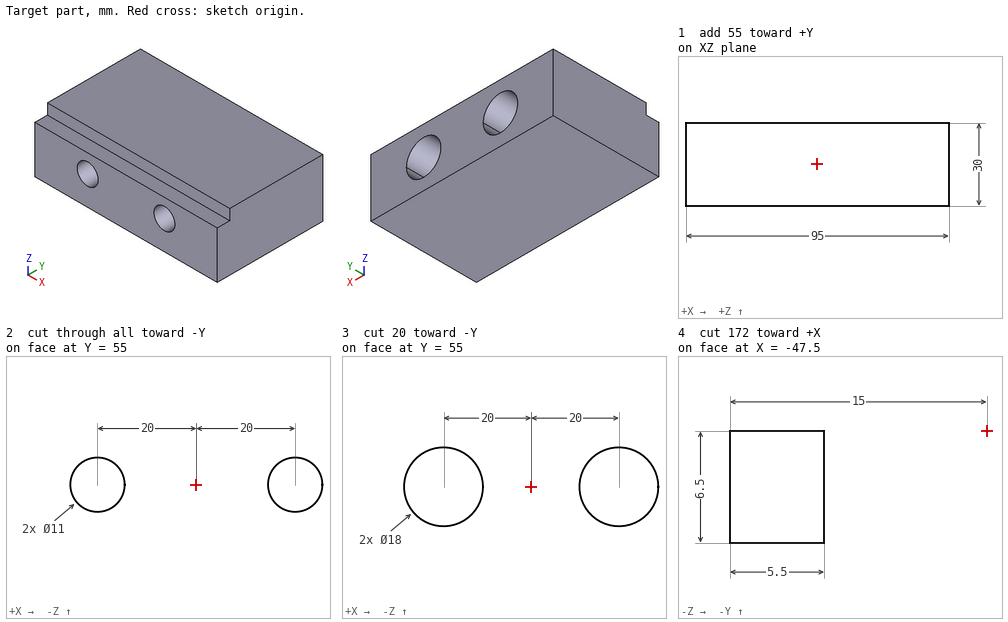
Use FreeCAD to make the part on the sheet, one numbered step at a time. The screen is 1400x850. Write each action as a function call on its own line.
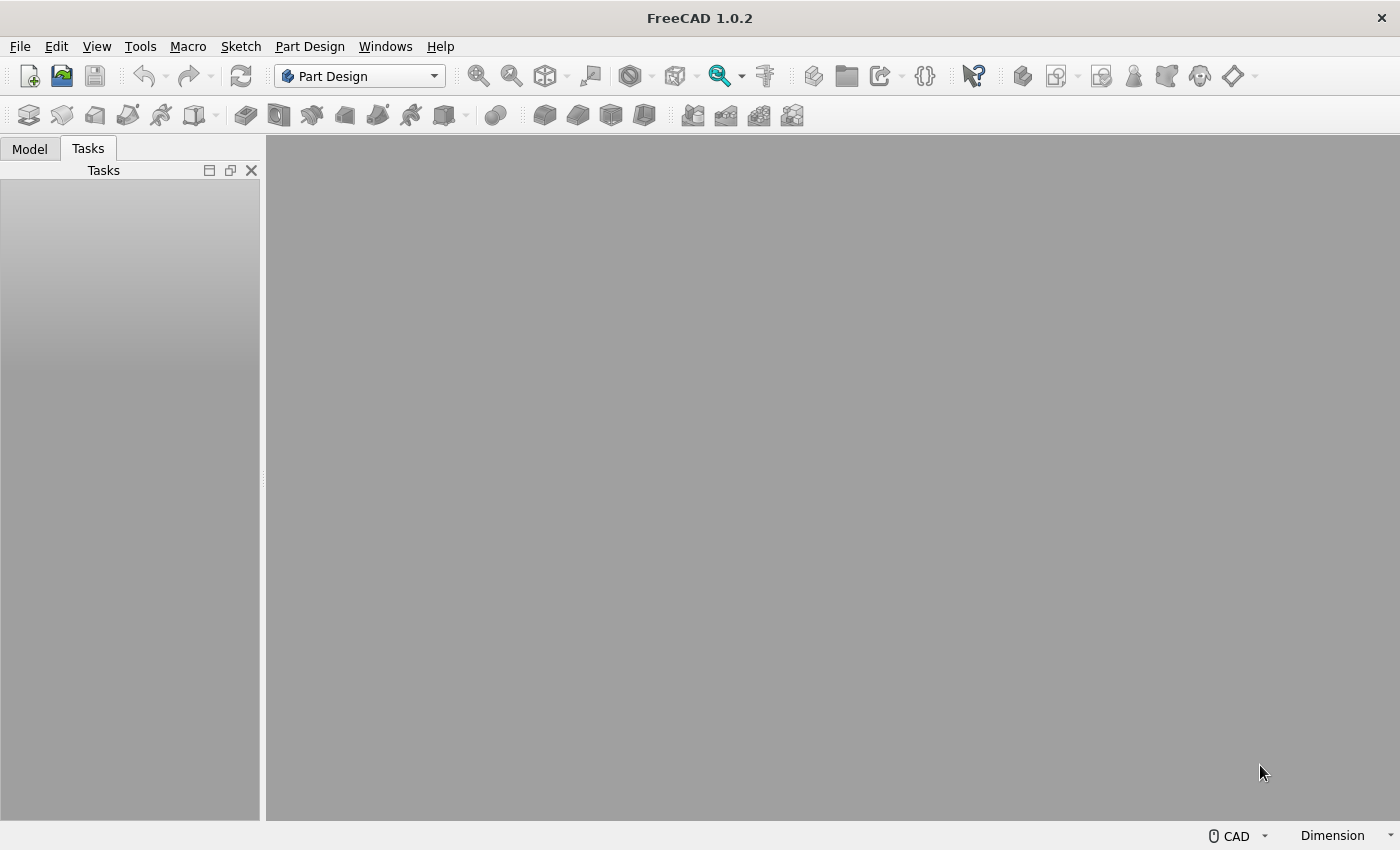
click(29, 76)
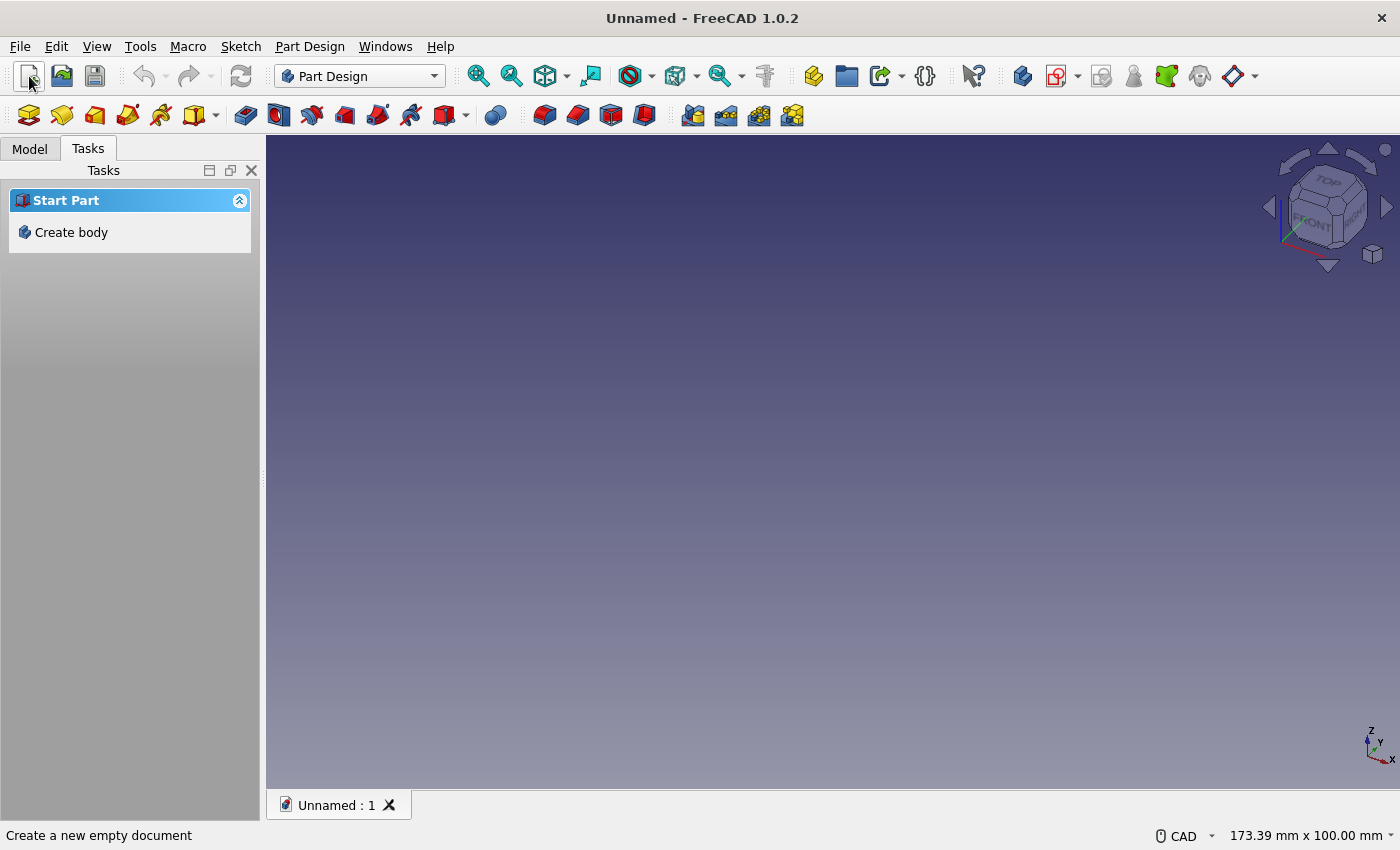
click(1056, 76)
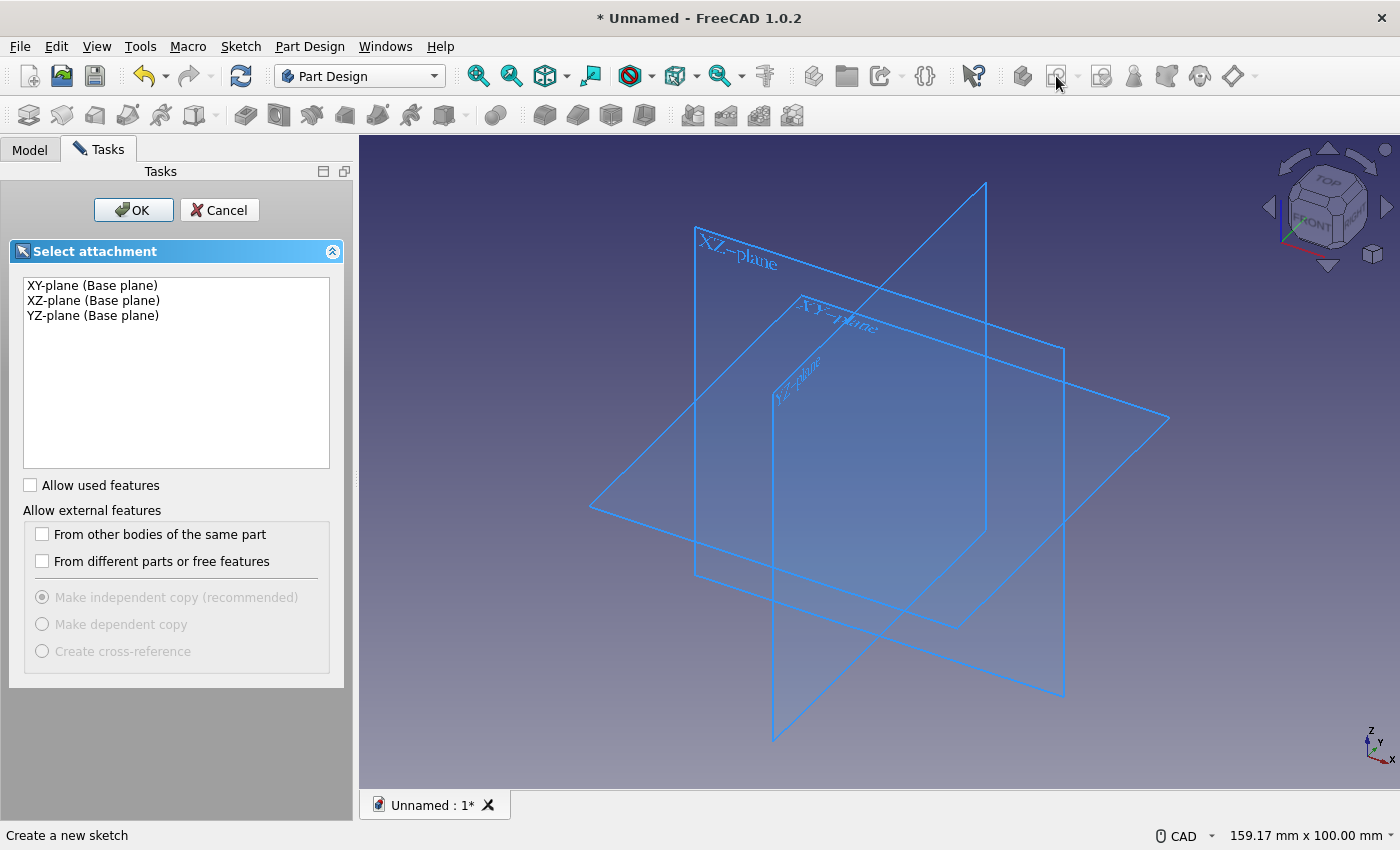
click(84, 300)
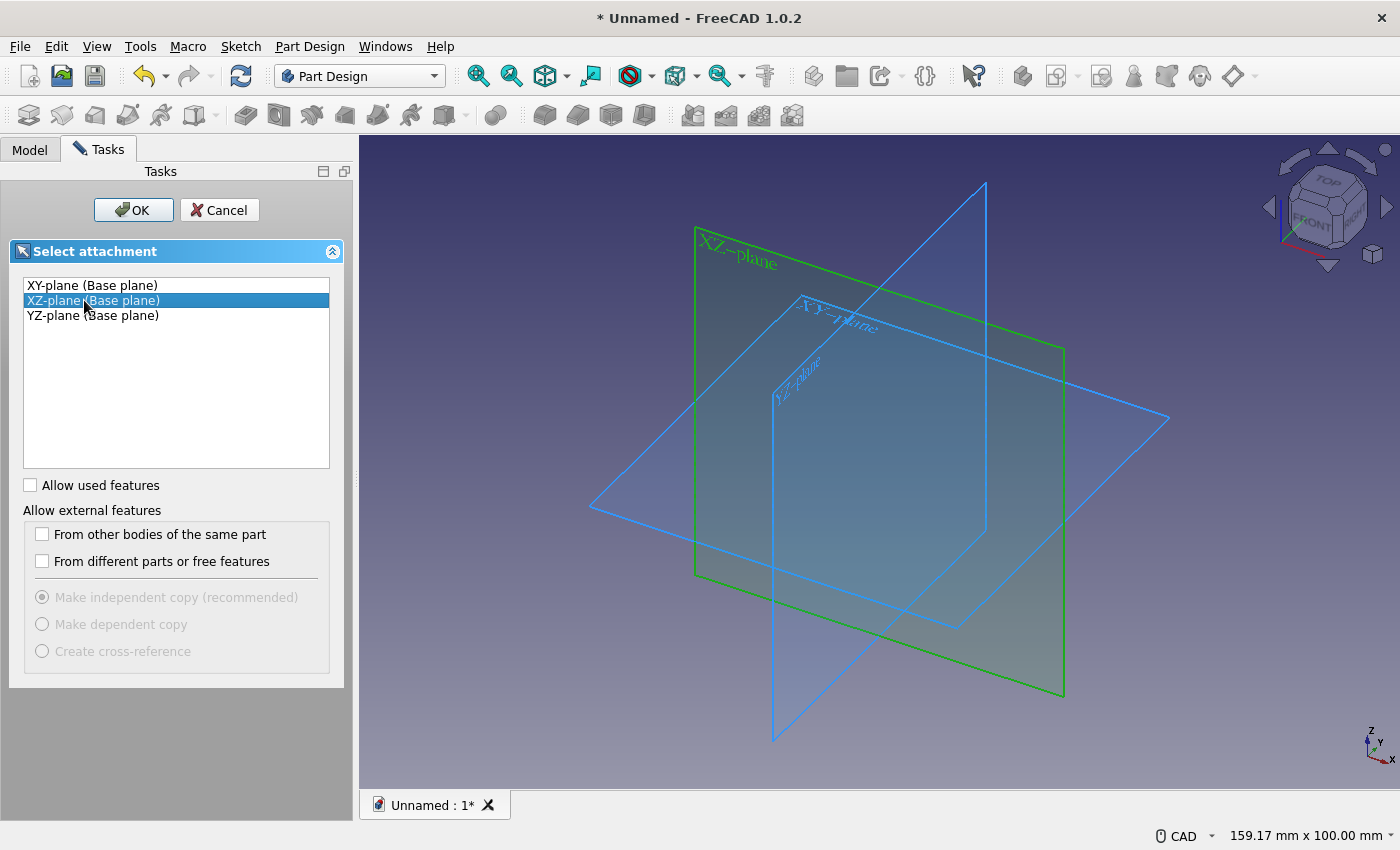
click(134, 210)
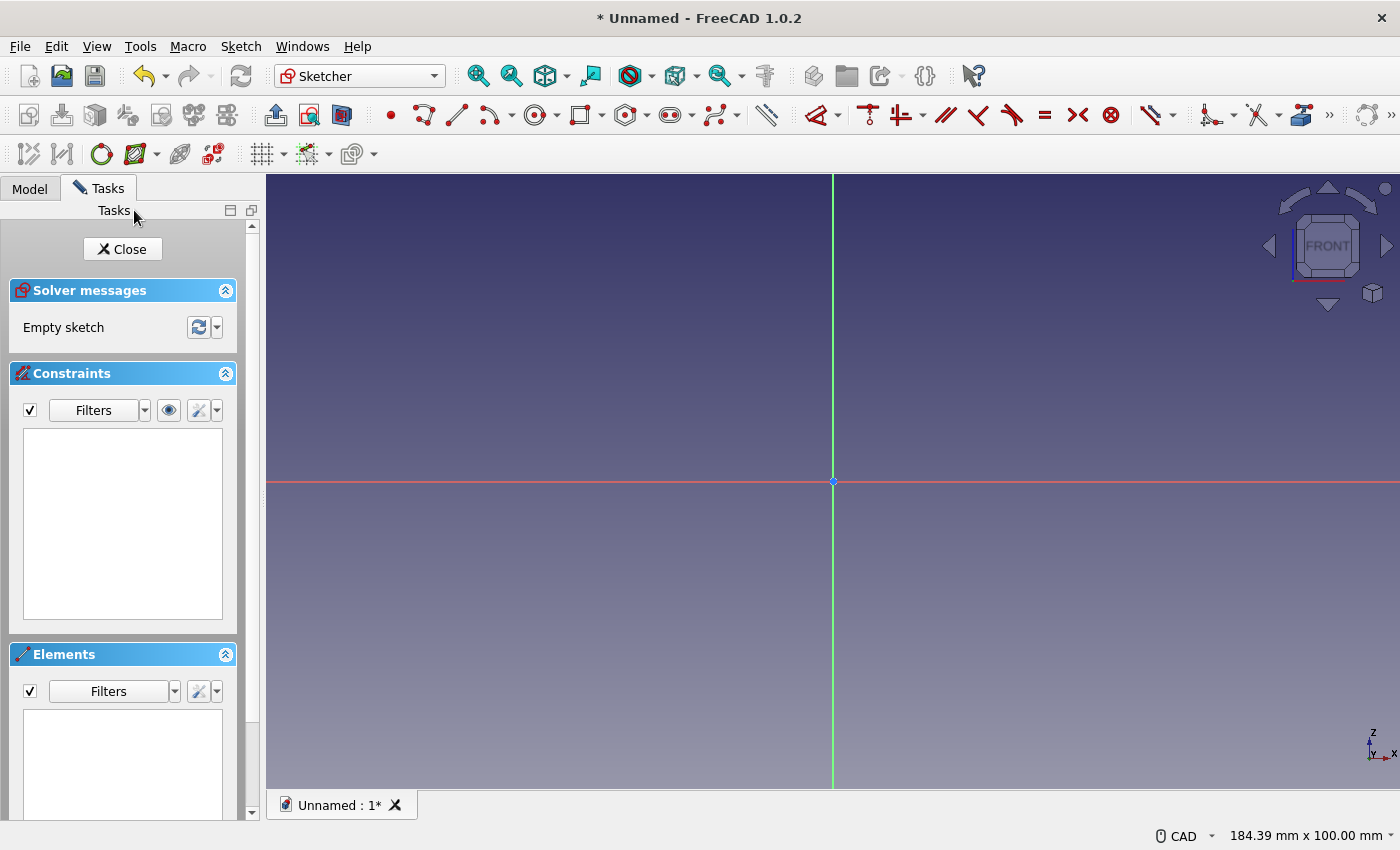
key(g)
key(v)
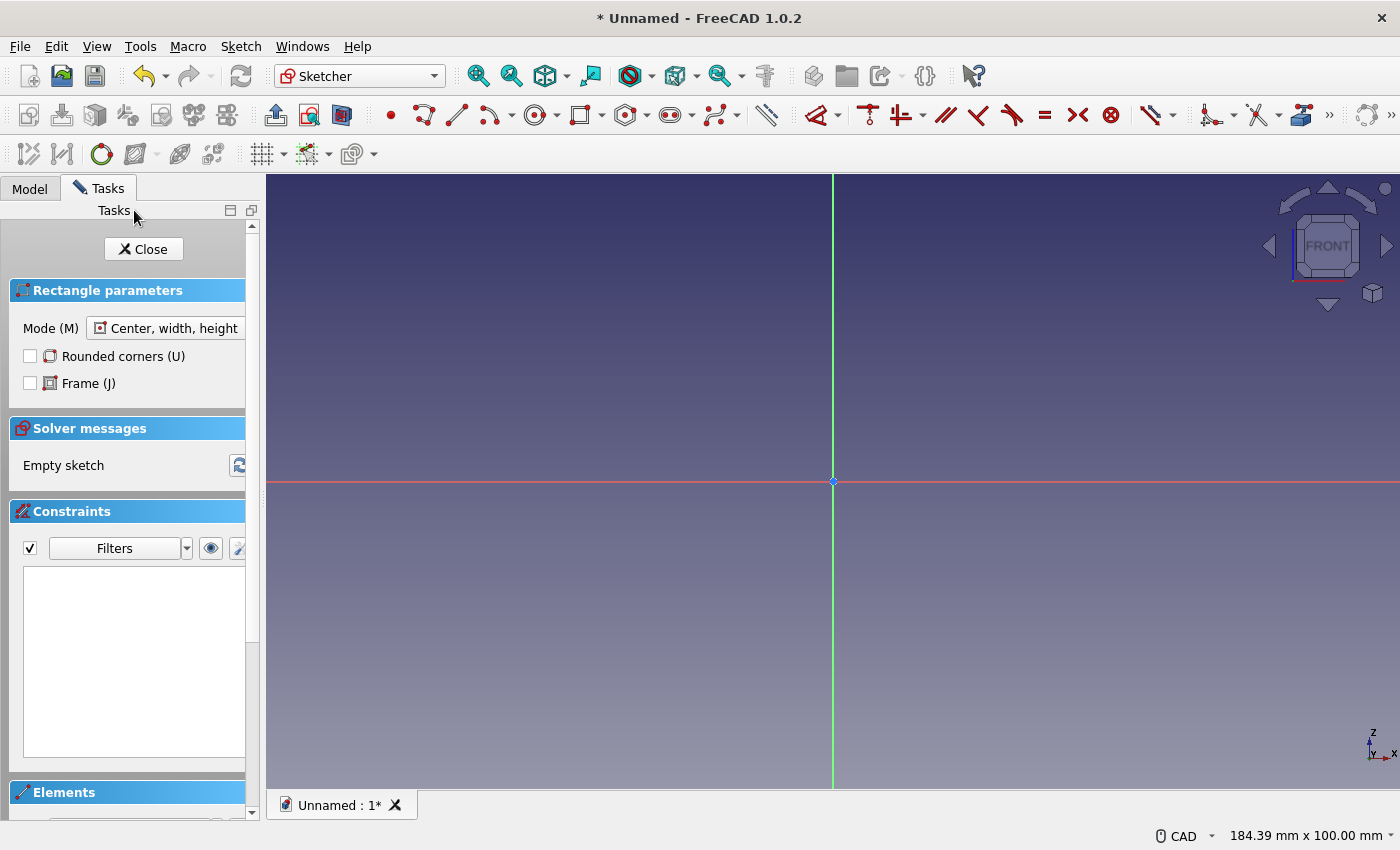
click(833, 482)
move(1125, 389)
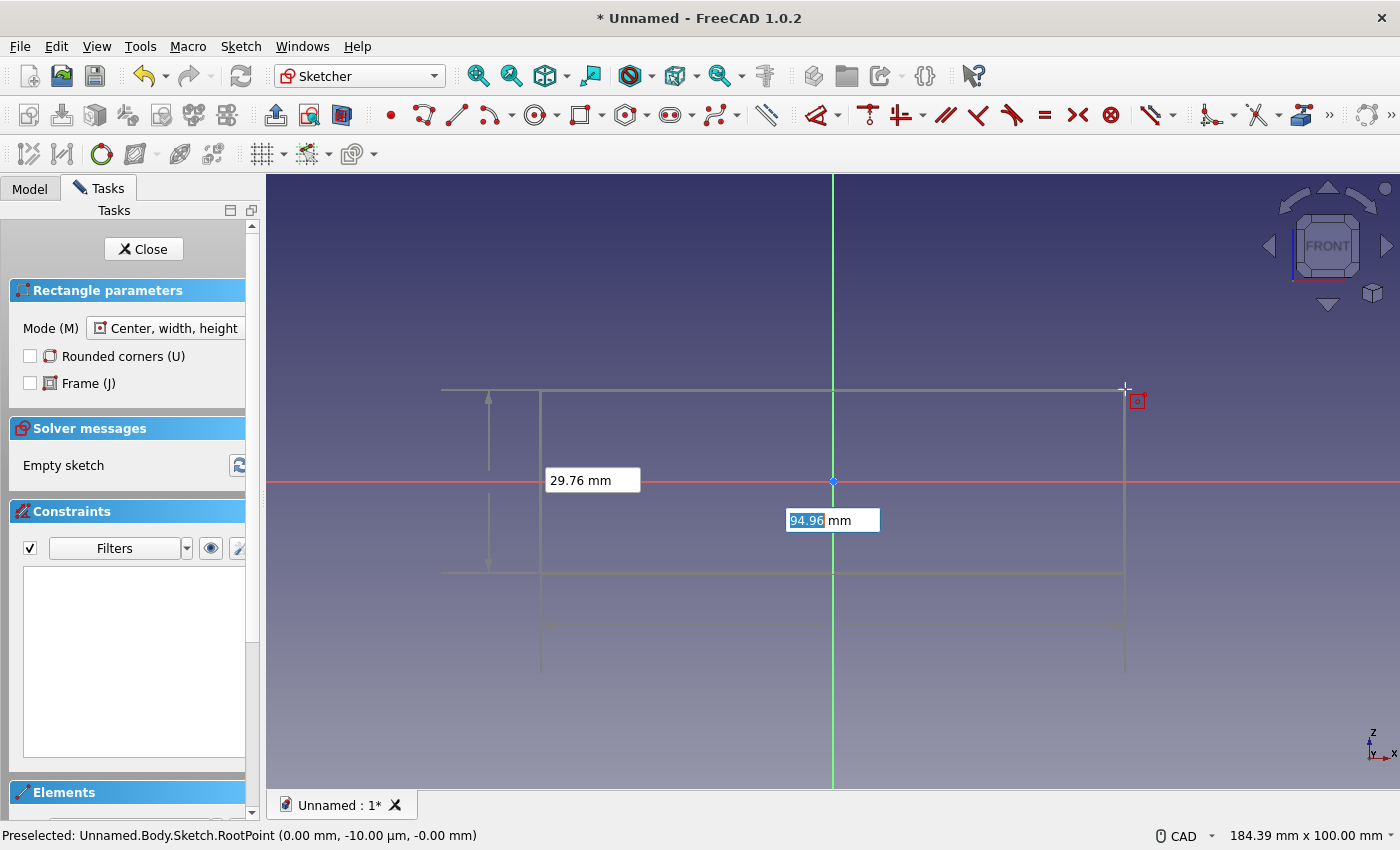
text(95)
key(Tab)
text(30)
key(Return)
key(Escape)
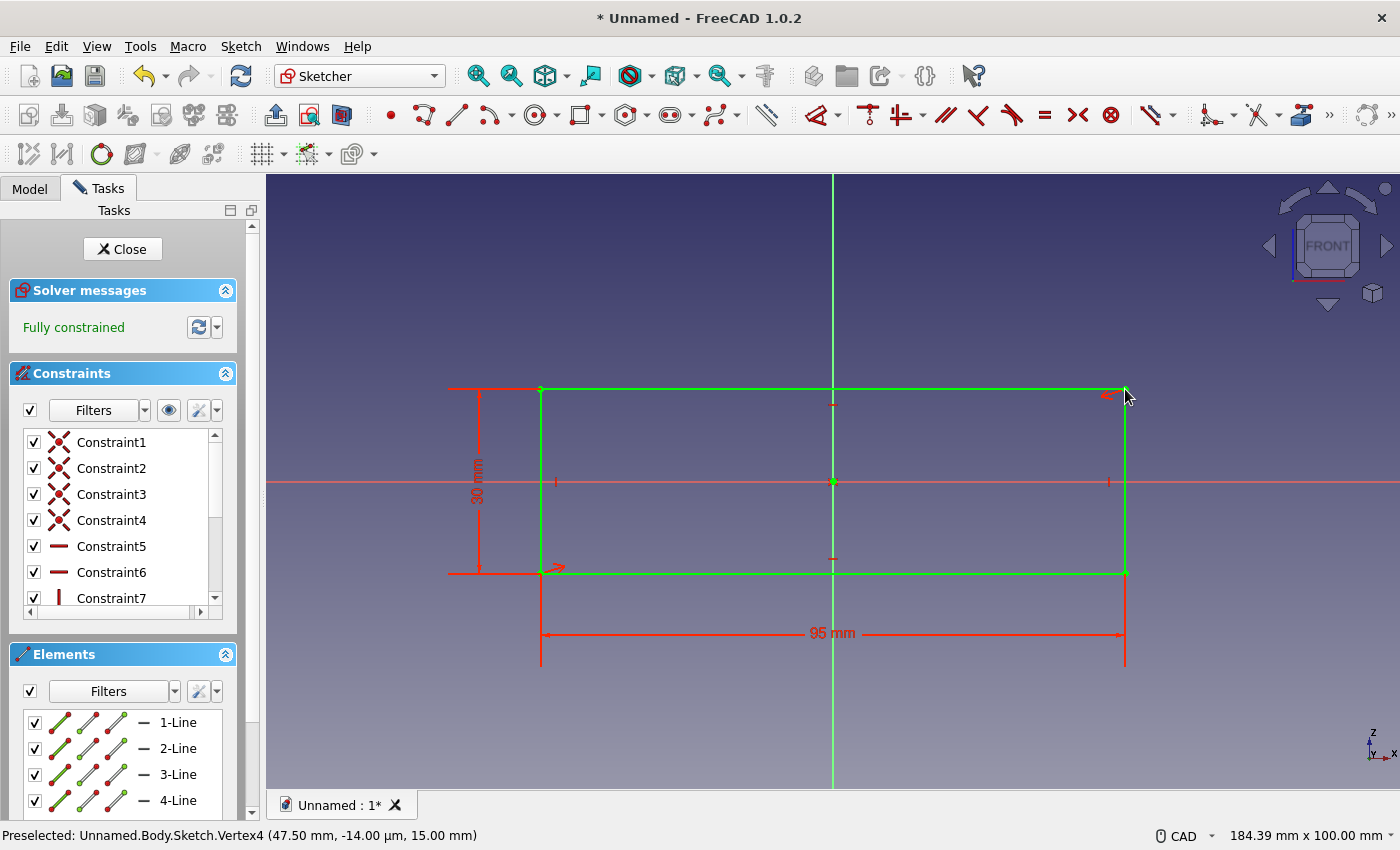
click(123, 249)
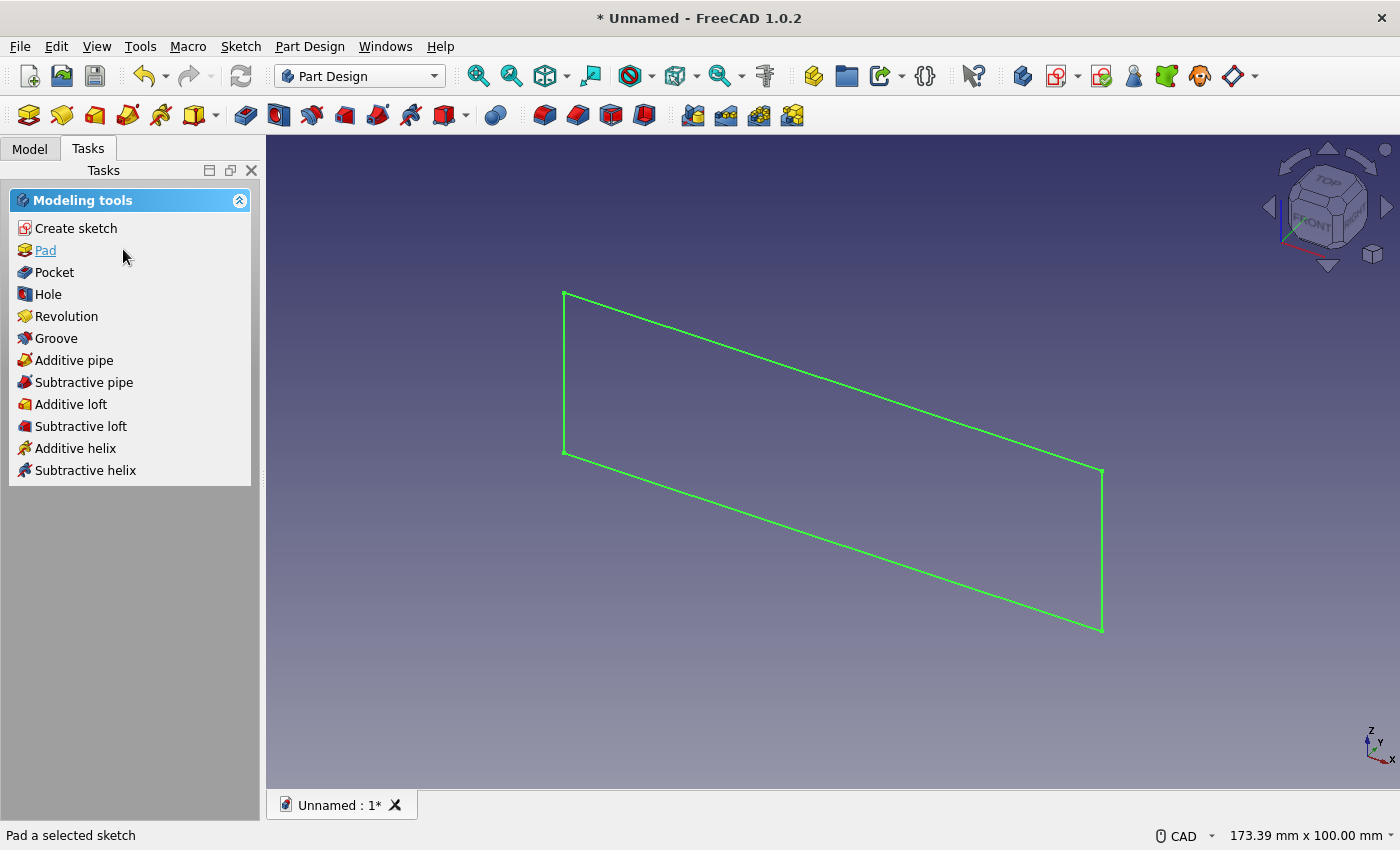
click(29, 116)